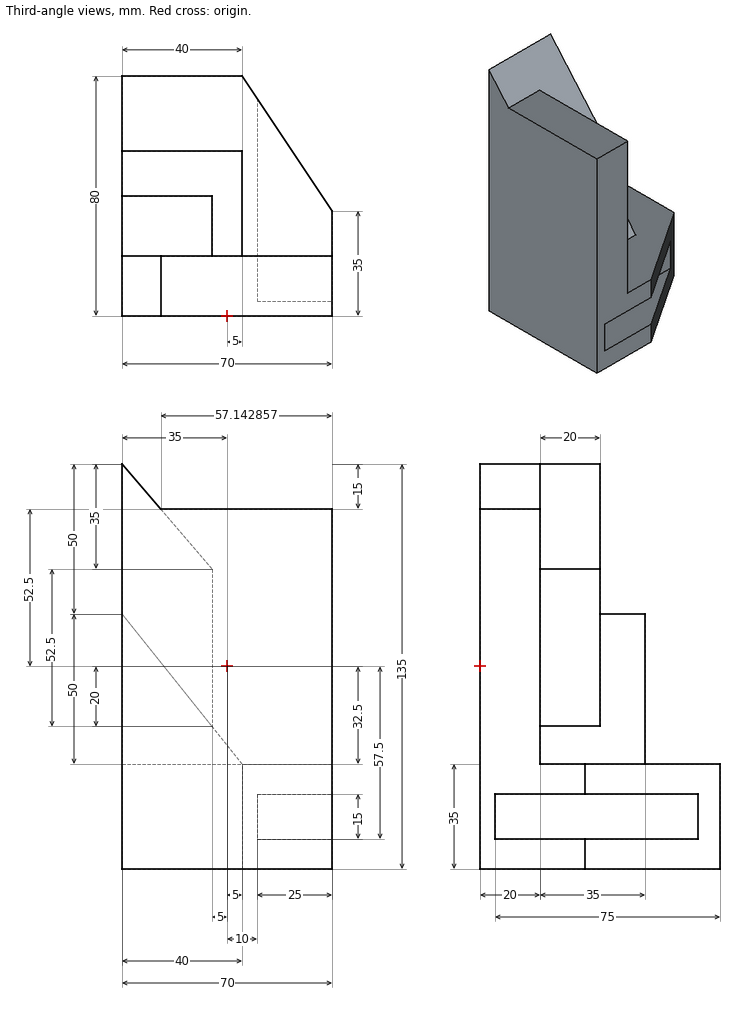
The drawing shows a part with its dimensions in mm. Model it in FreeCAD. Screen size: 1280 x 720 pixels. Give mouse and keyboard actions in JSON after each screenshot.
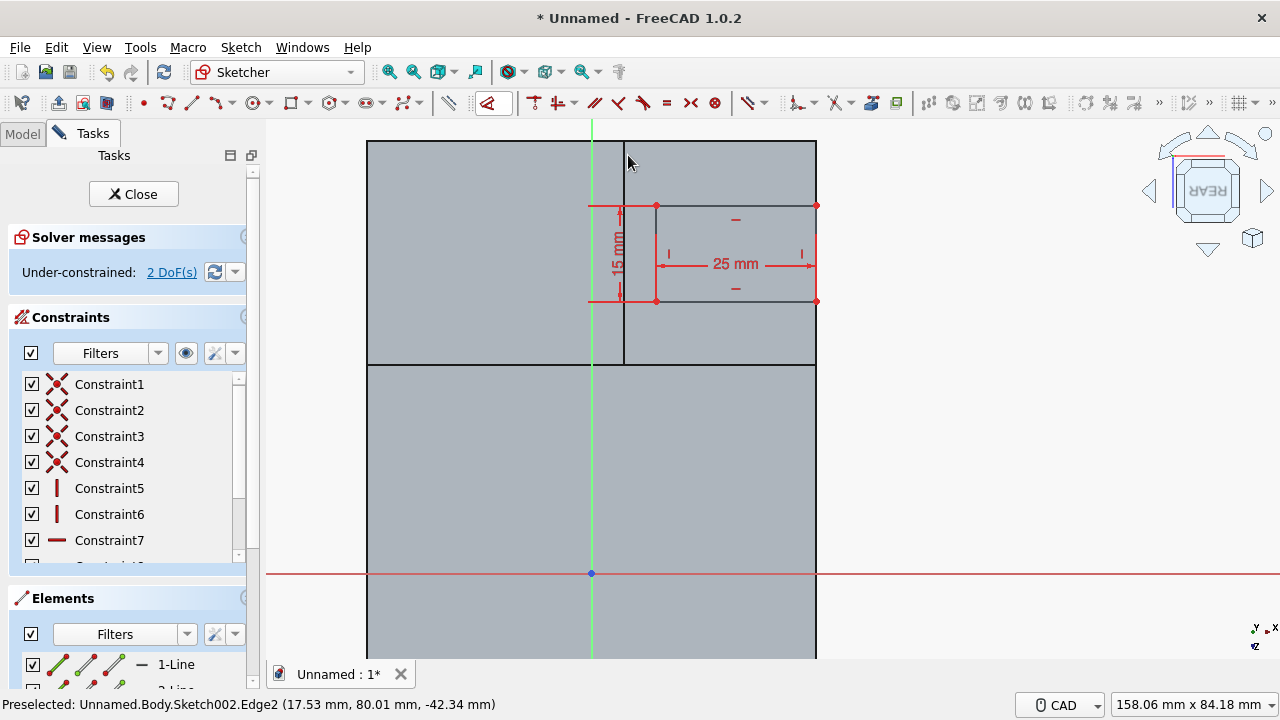
{"action": "left_click", "coordinate": [656, 206]}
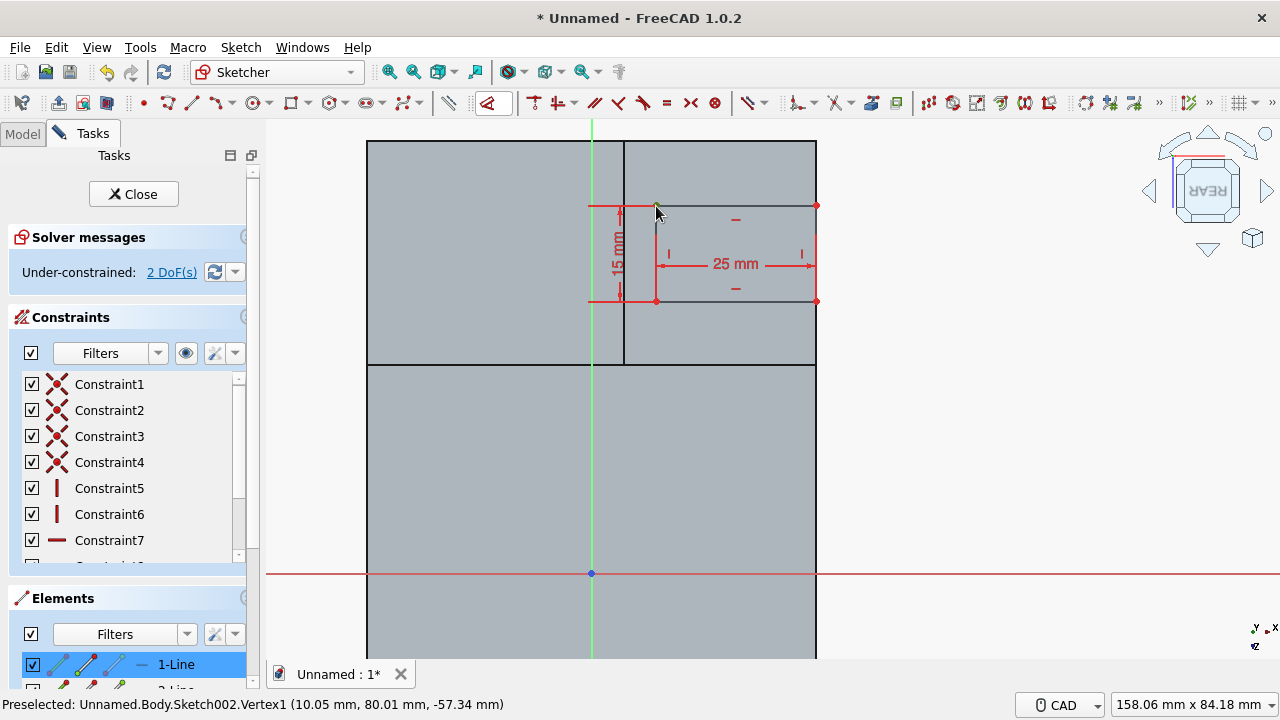
{"action": "key", "text": "l"}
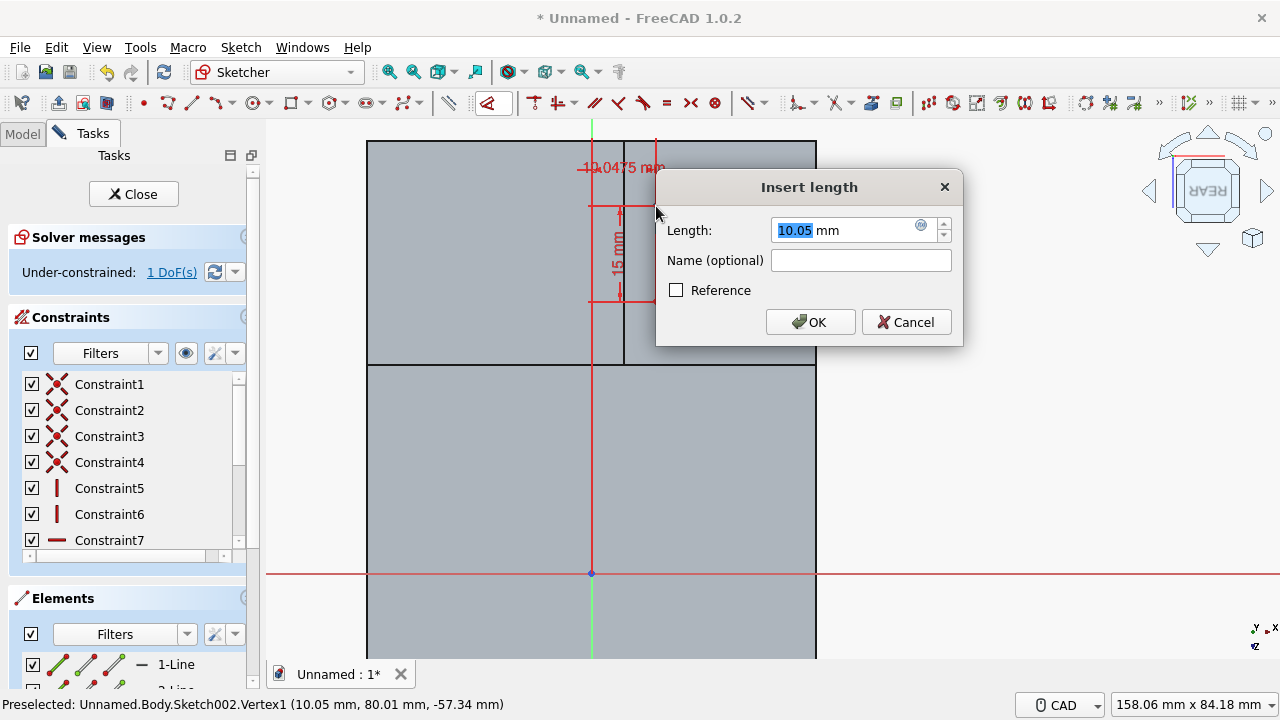
{"action": "type", "text": "10"}
{"action": "key", "text": "Return"}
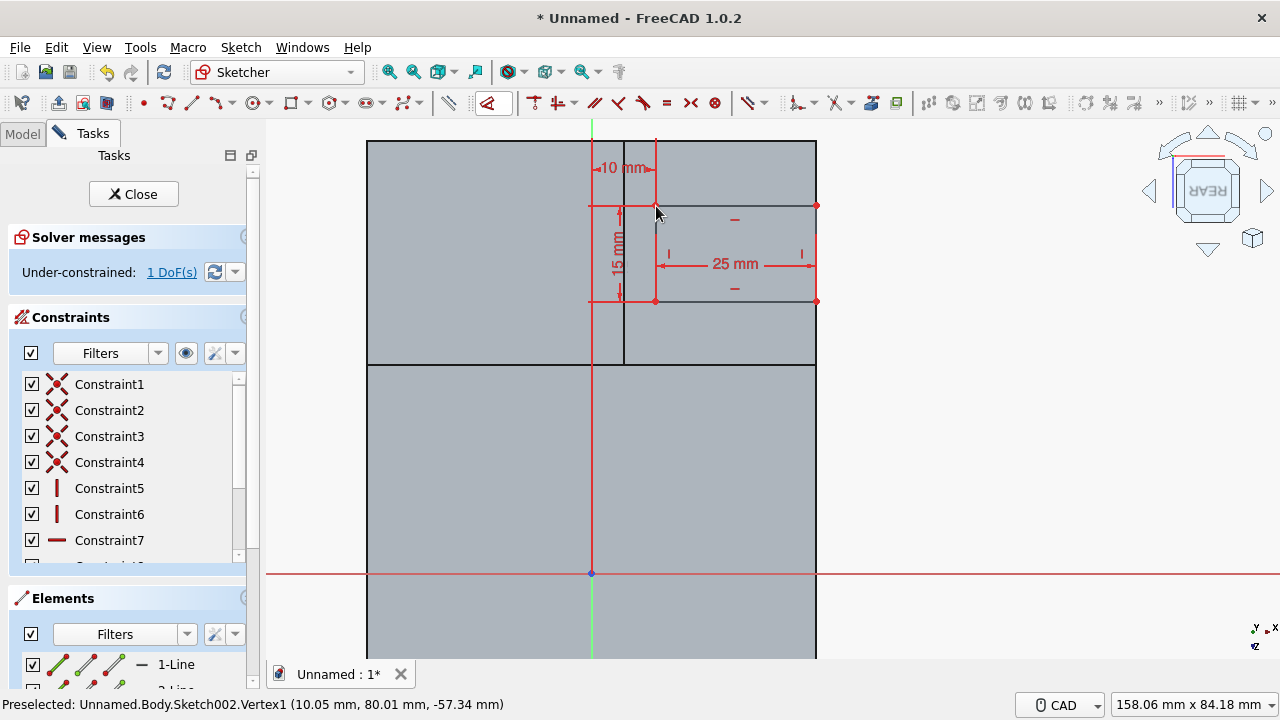
{"action": "left_click", "coordinate": [656, 206]}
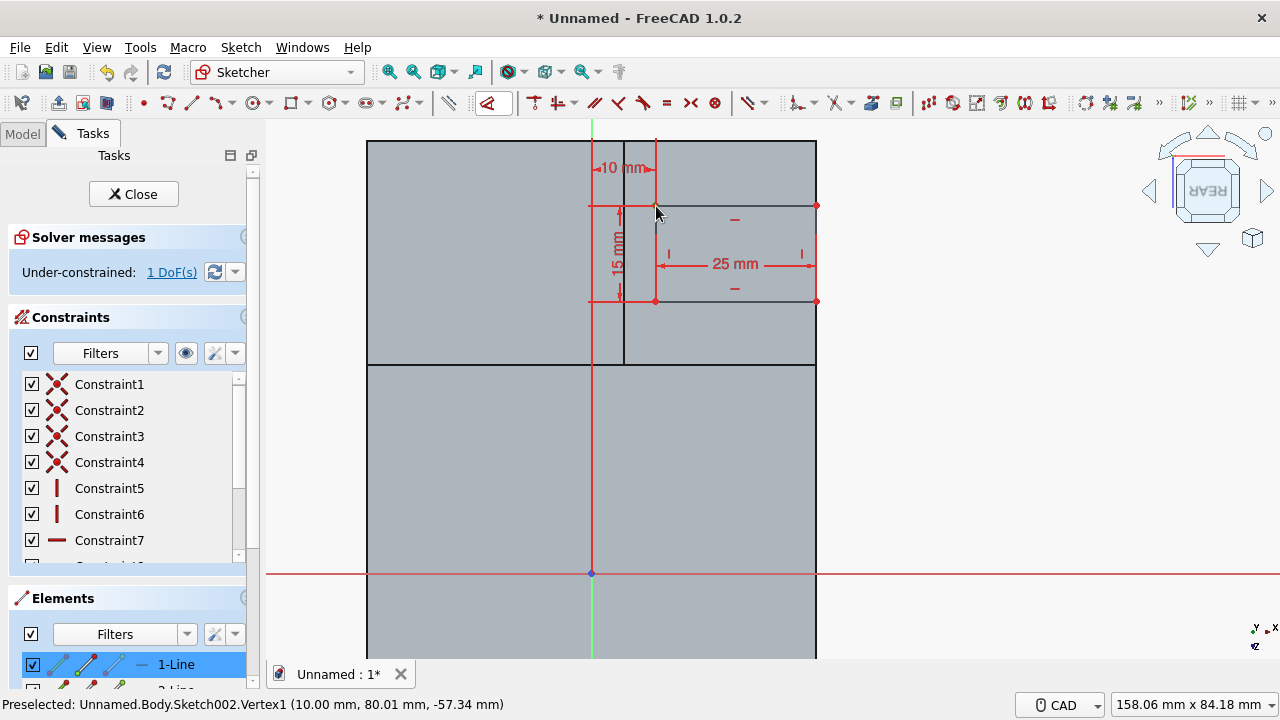
{"action": "left_click", "coordinate": [506, 104]}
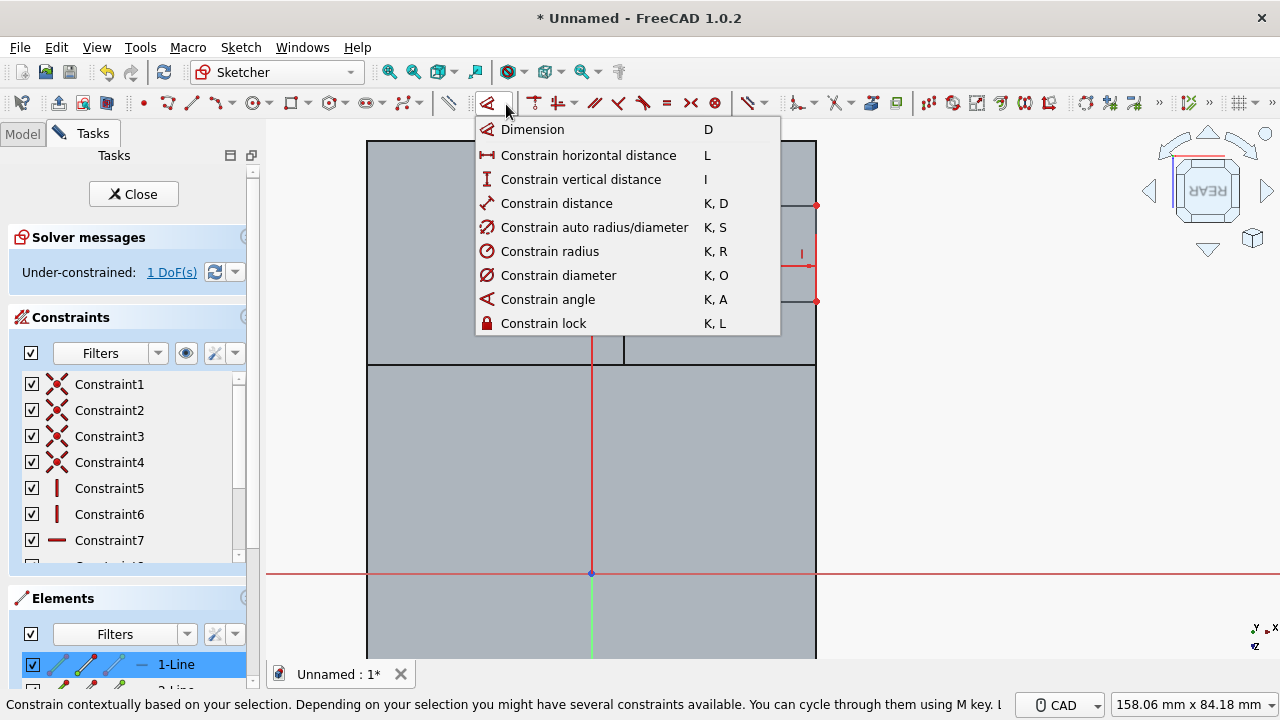
{"action": "left_click", "coordinate": [628, 179]}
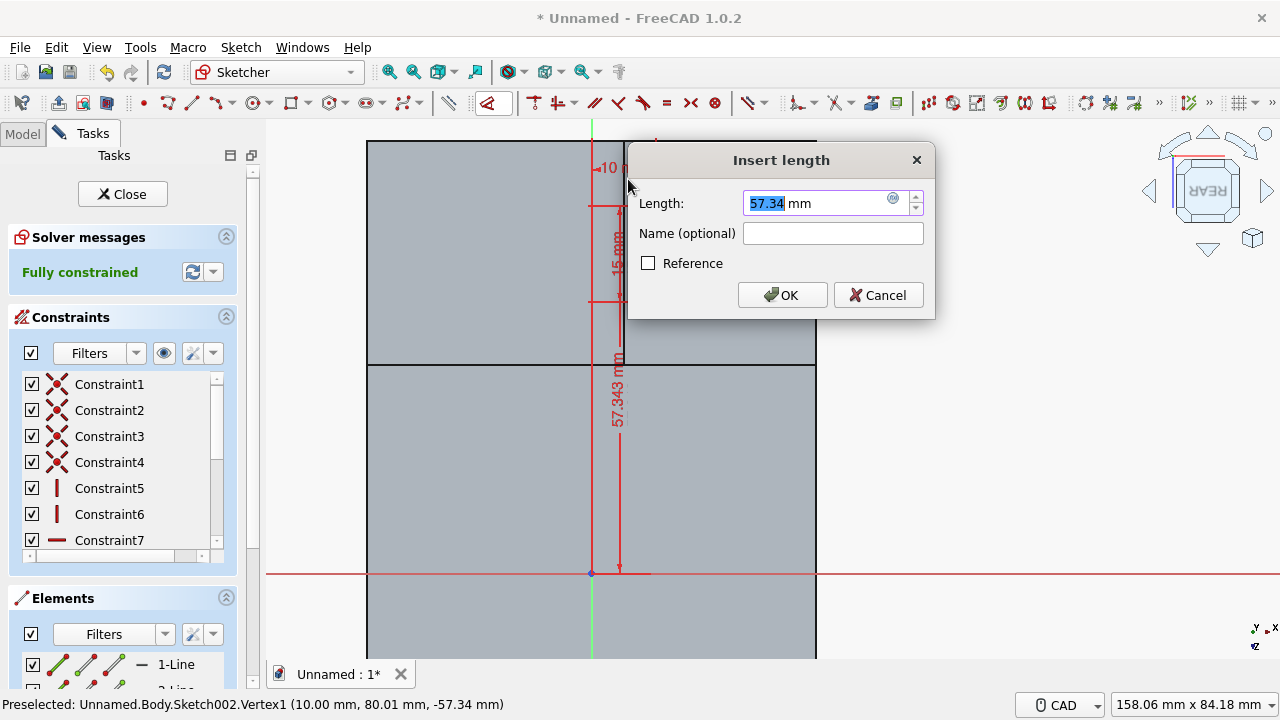
{"action": "type", "text": "57.5"}
{"action": "key", "text": "Return"}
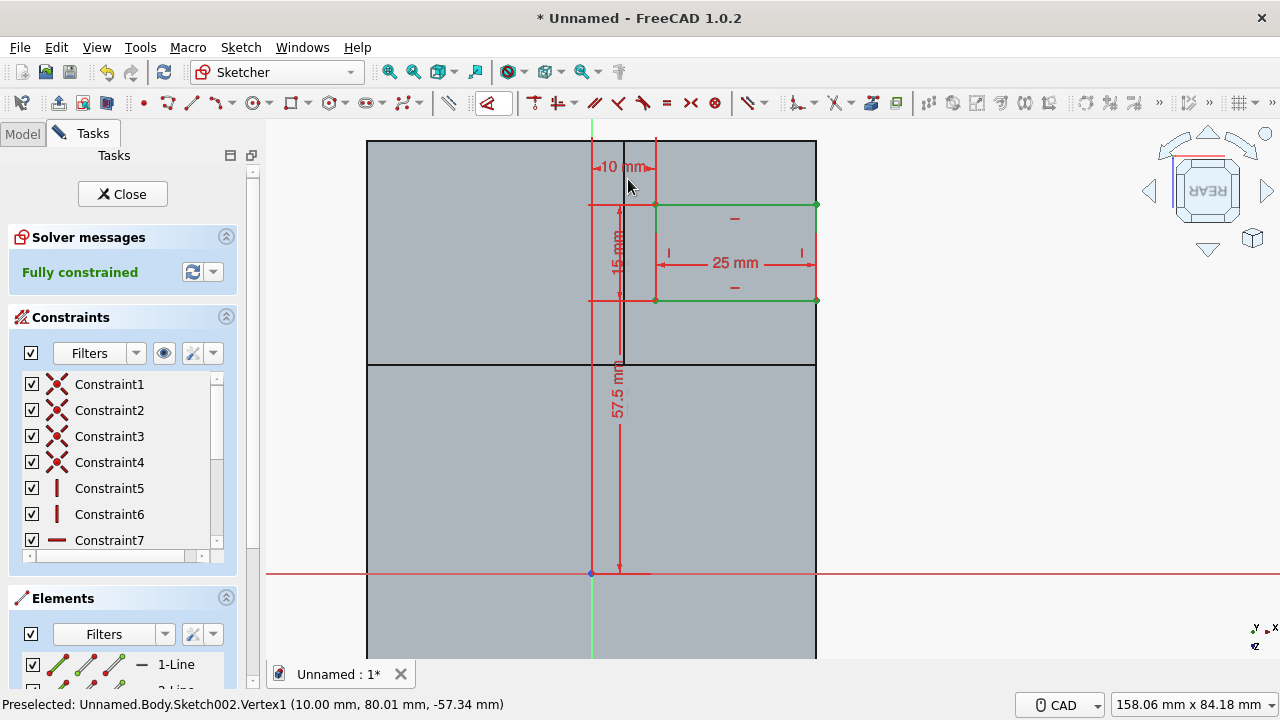
{"action": "left_click", "coordinate": [123, 194]}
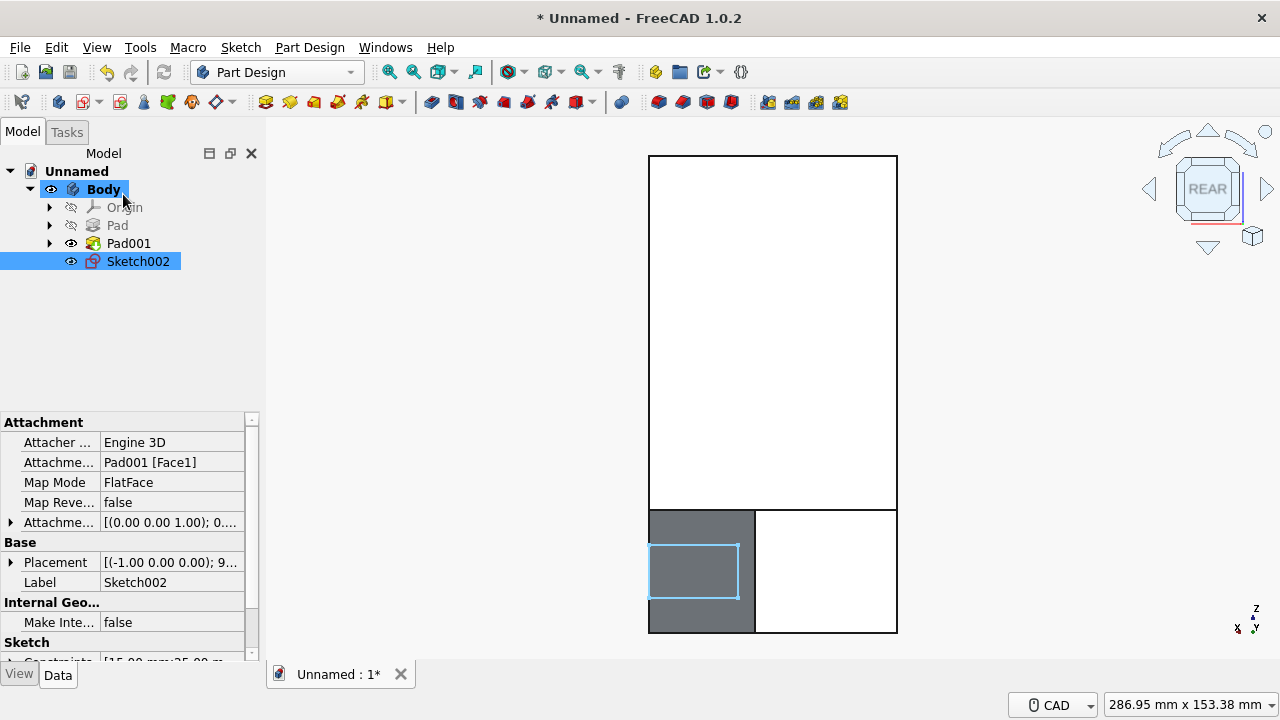
{"action": "left_click", "coordinate": [432, 102]}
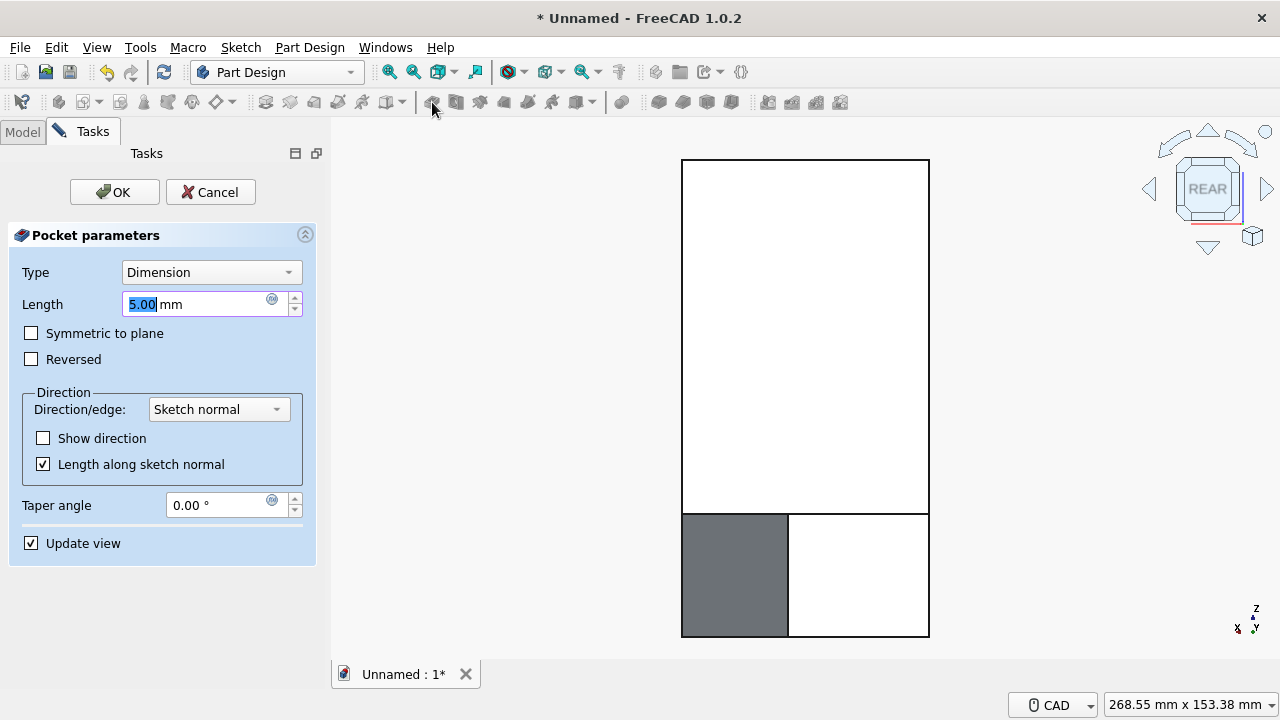
{"action": "type", "text": "75"}
{"action": "key", "text": "Tab"}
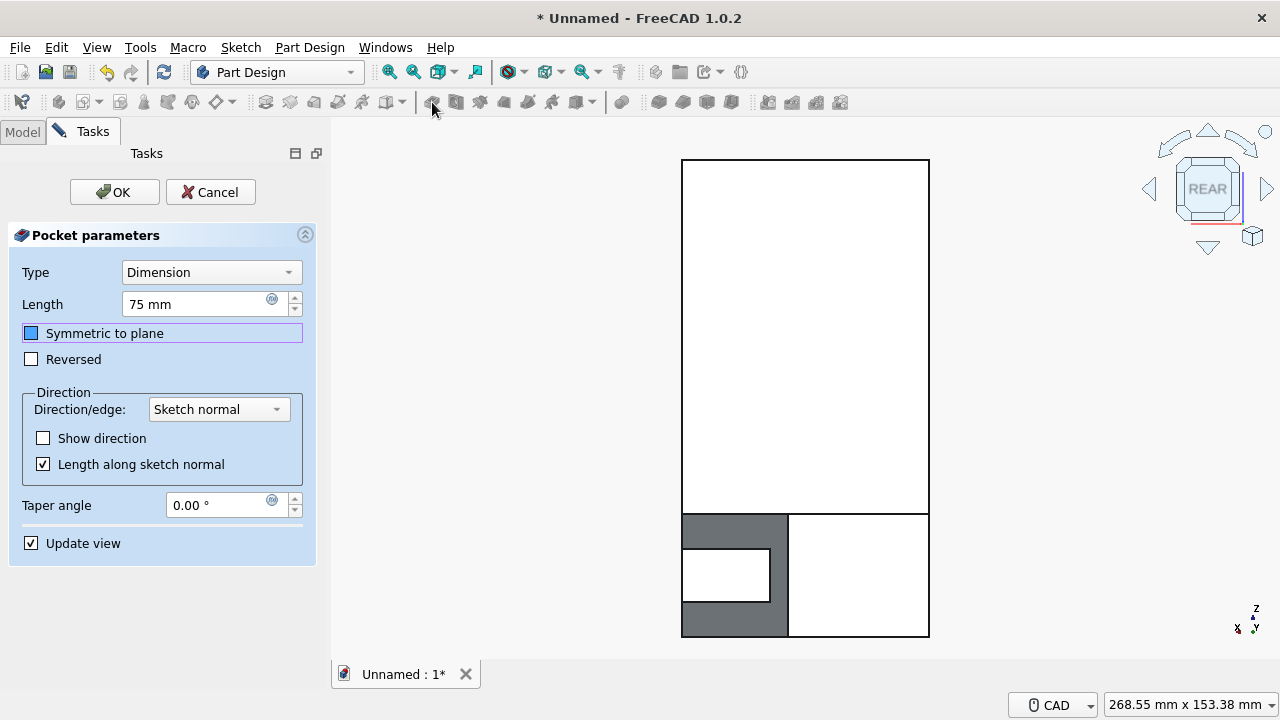
{"action": "left_click", "coordinate": [115, 192]}